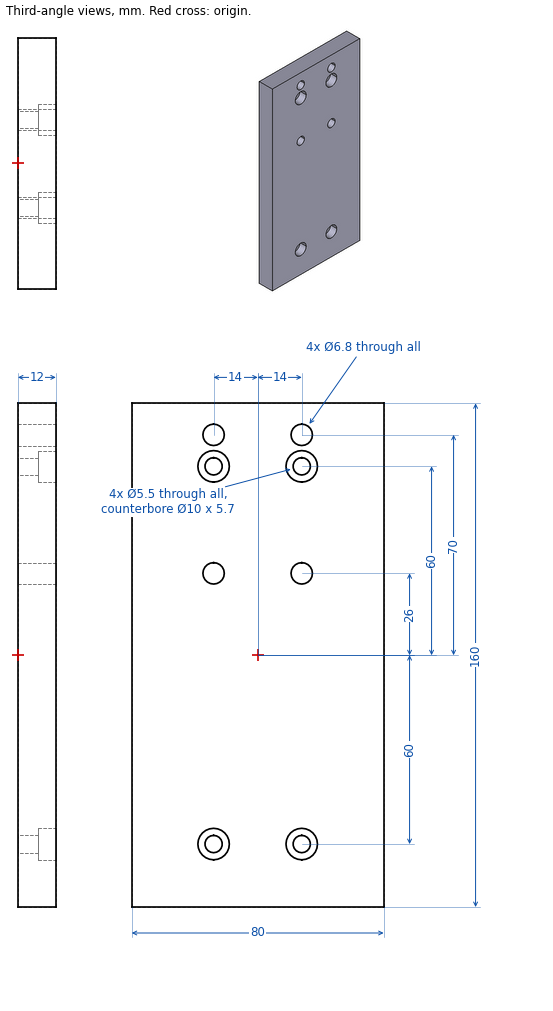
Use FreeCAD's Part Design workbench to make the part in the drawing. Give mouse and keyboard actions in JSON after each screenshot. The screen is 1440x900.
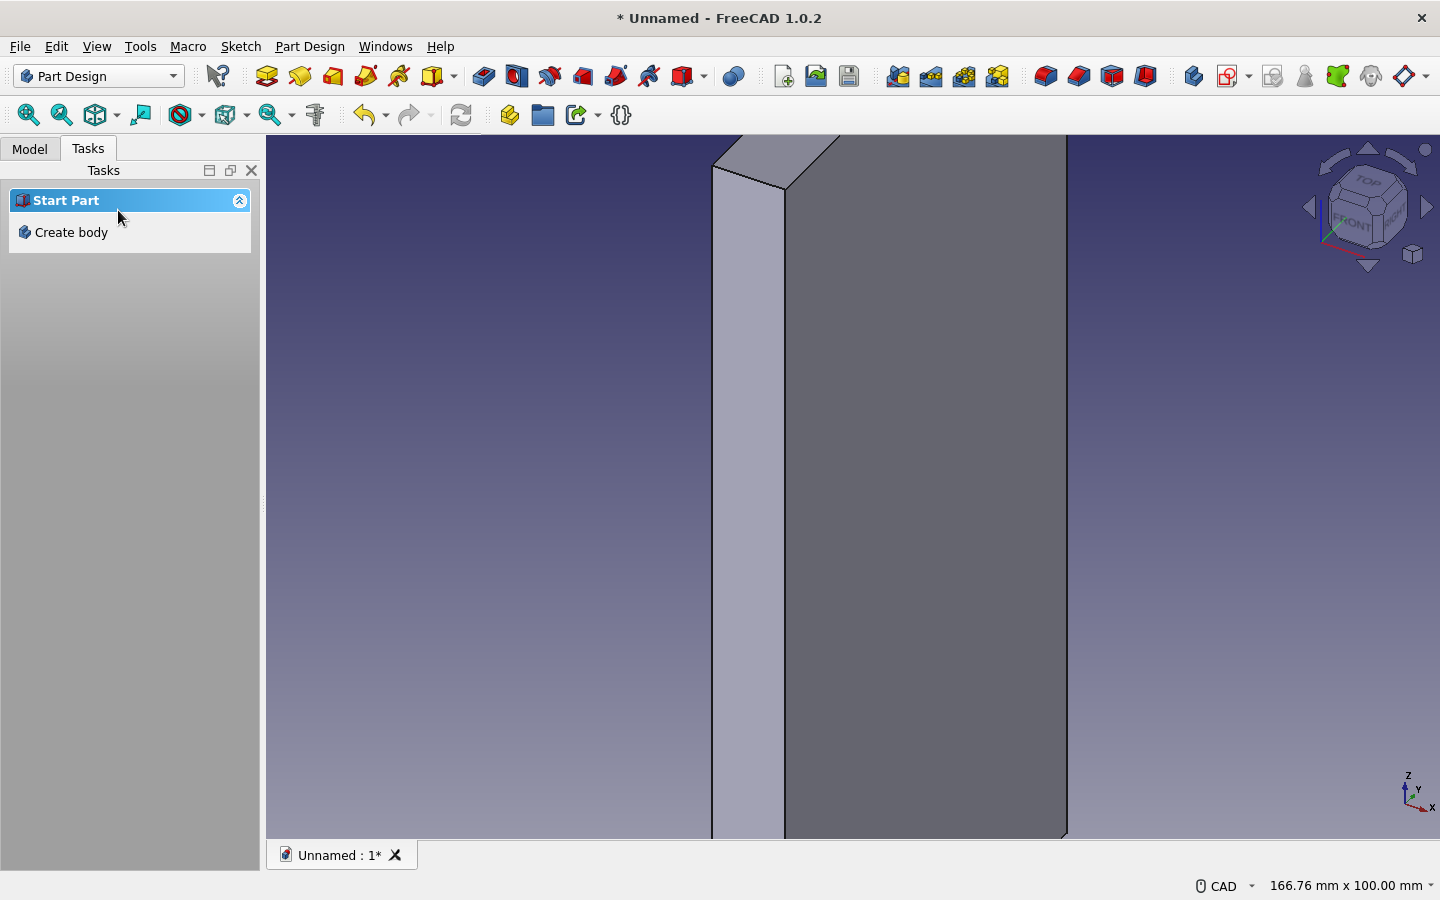
{"action": "left_click", "coordinate": [29, 116]}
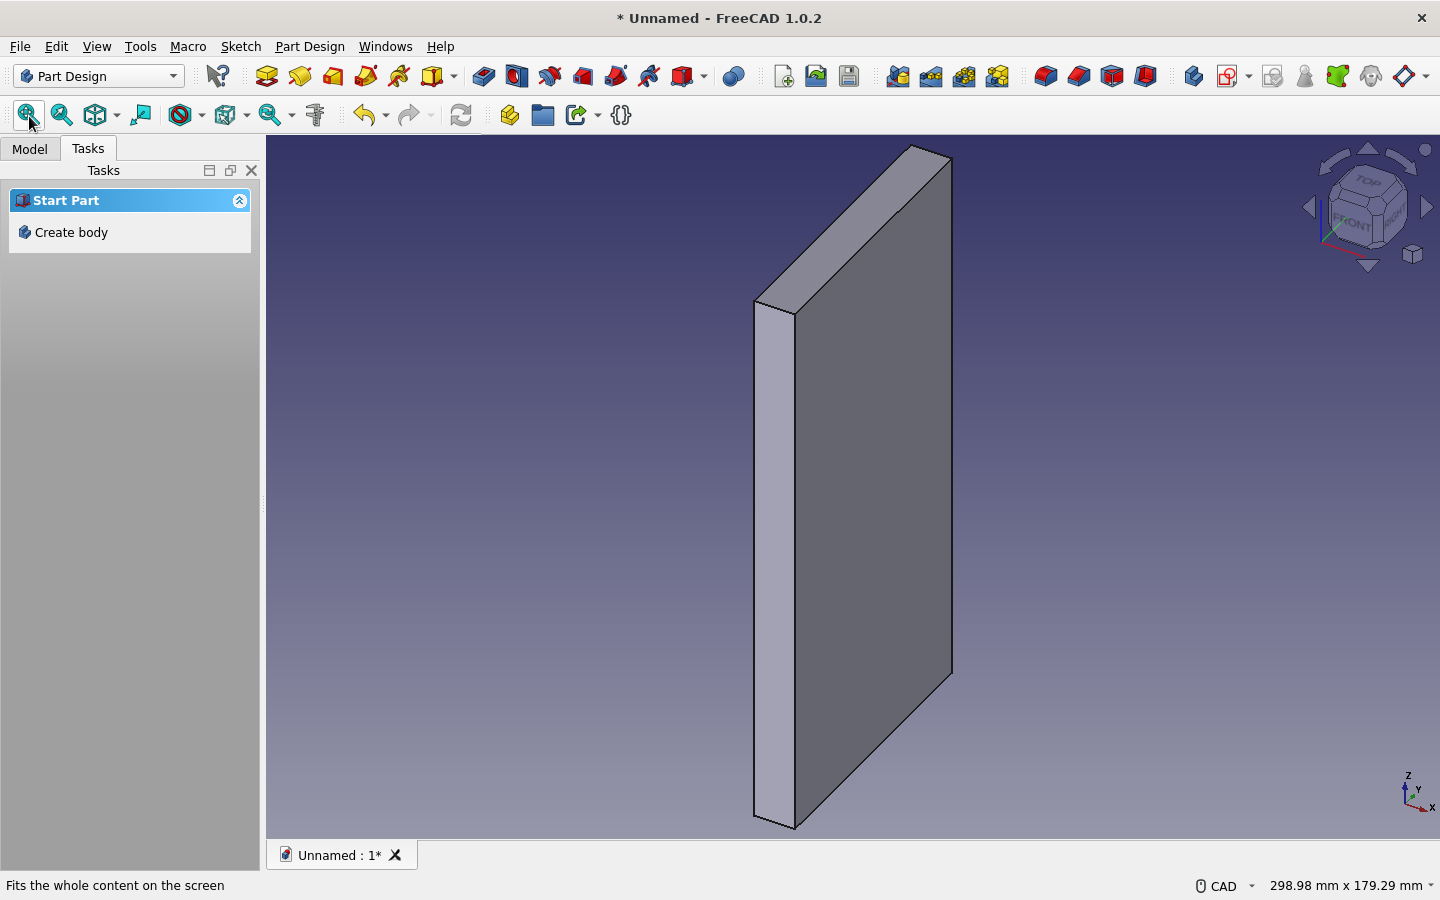
{"action": "left_click", "coordinate": [873, 566]}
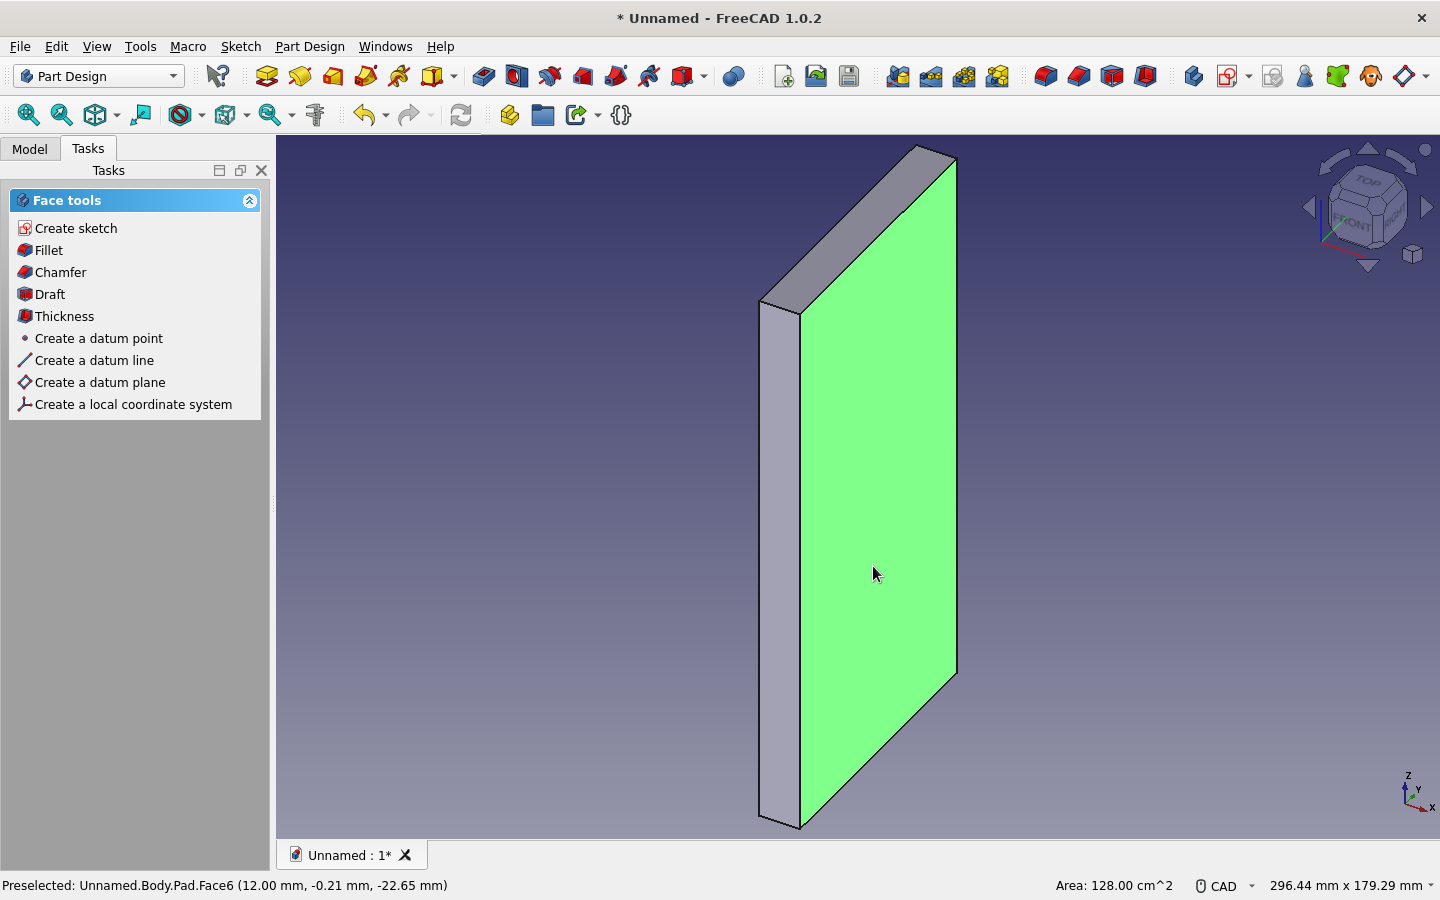
{"action": "left_click", "coordinate": [1226, 76]}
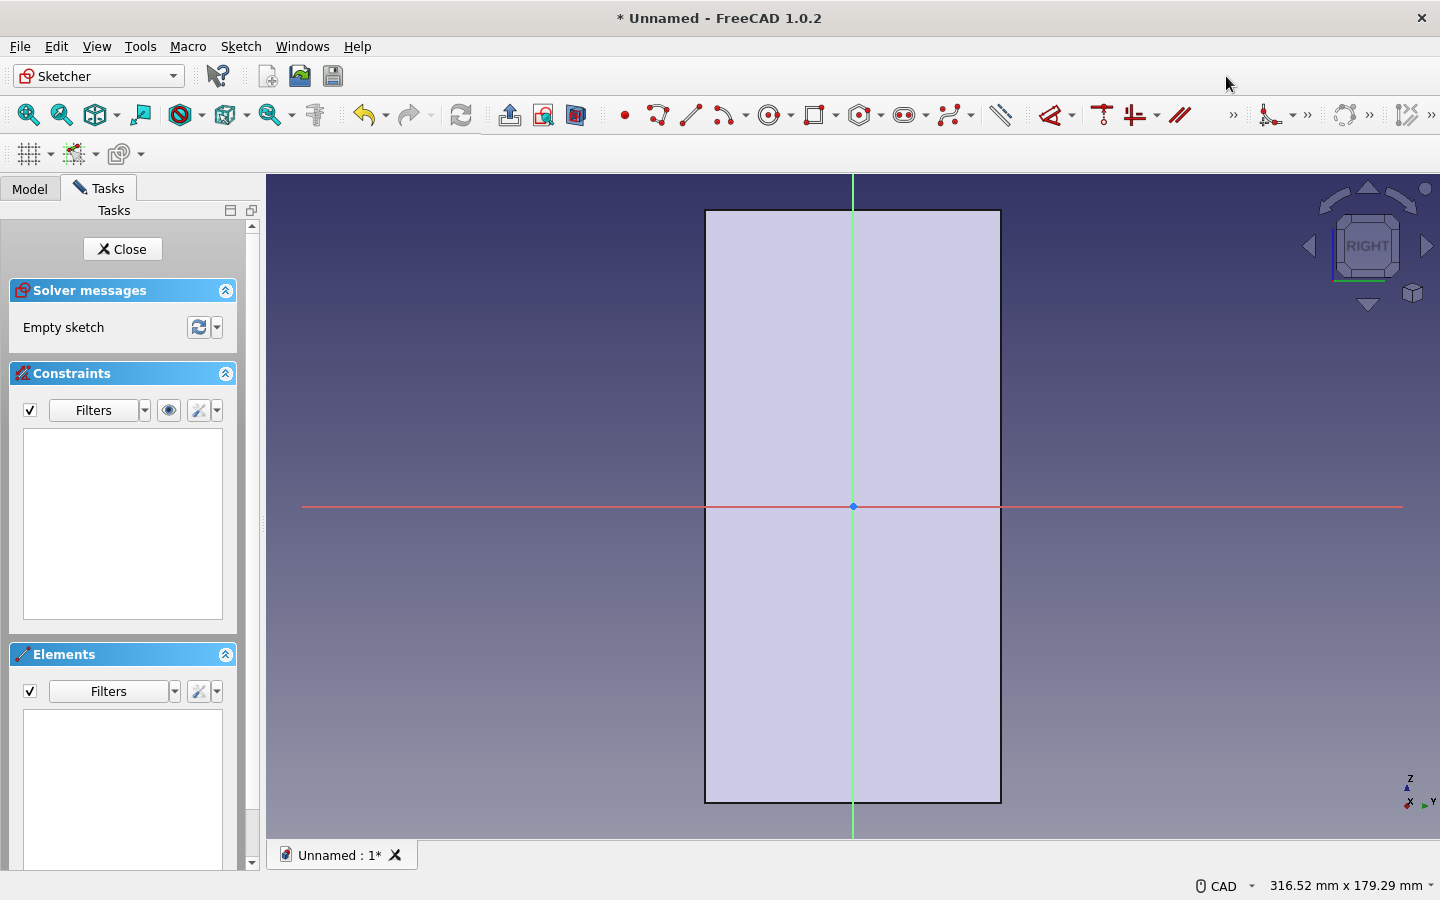
{"action": "scroll", "coordinate": [992, 202], "scroll_direction": "up", "scroll_amount": 2}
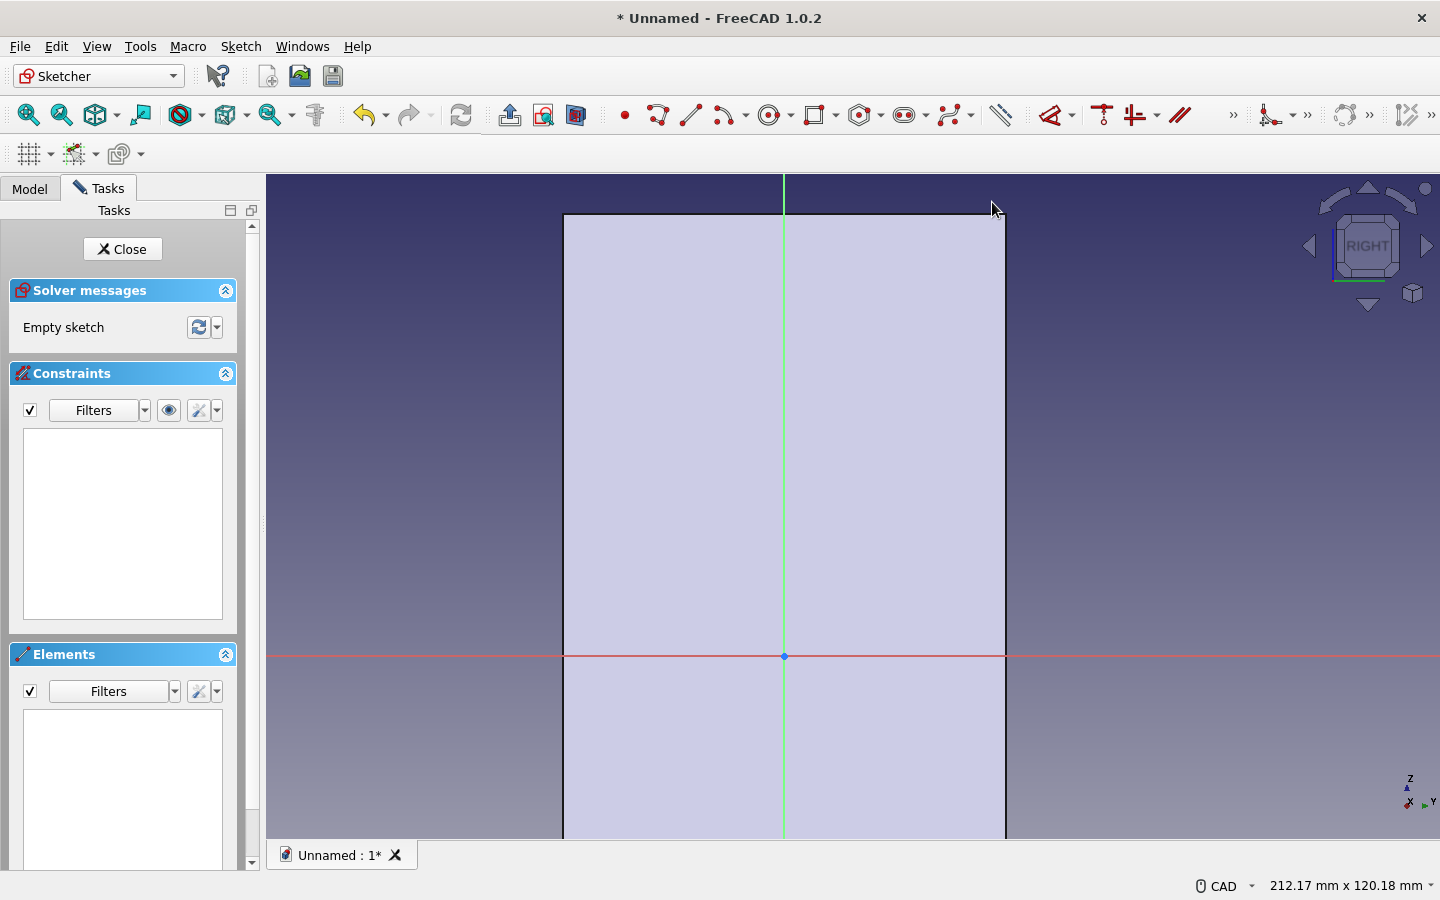
{"action": "left_click", "coordinate": [768, 116]}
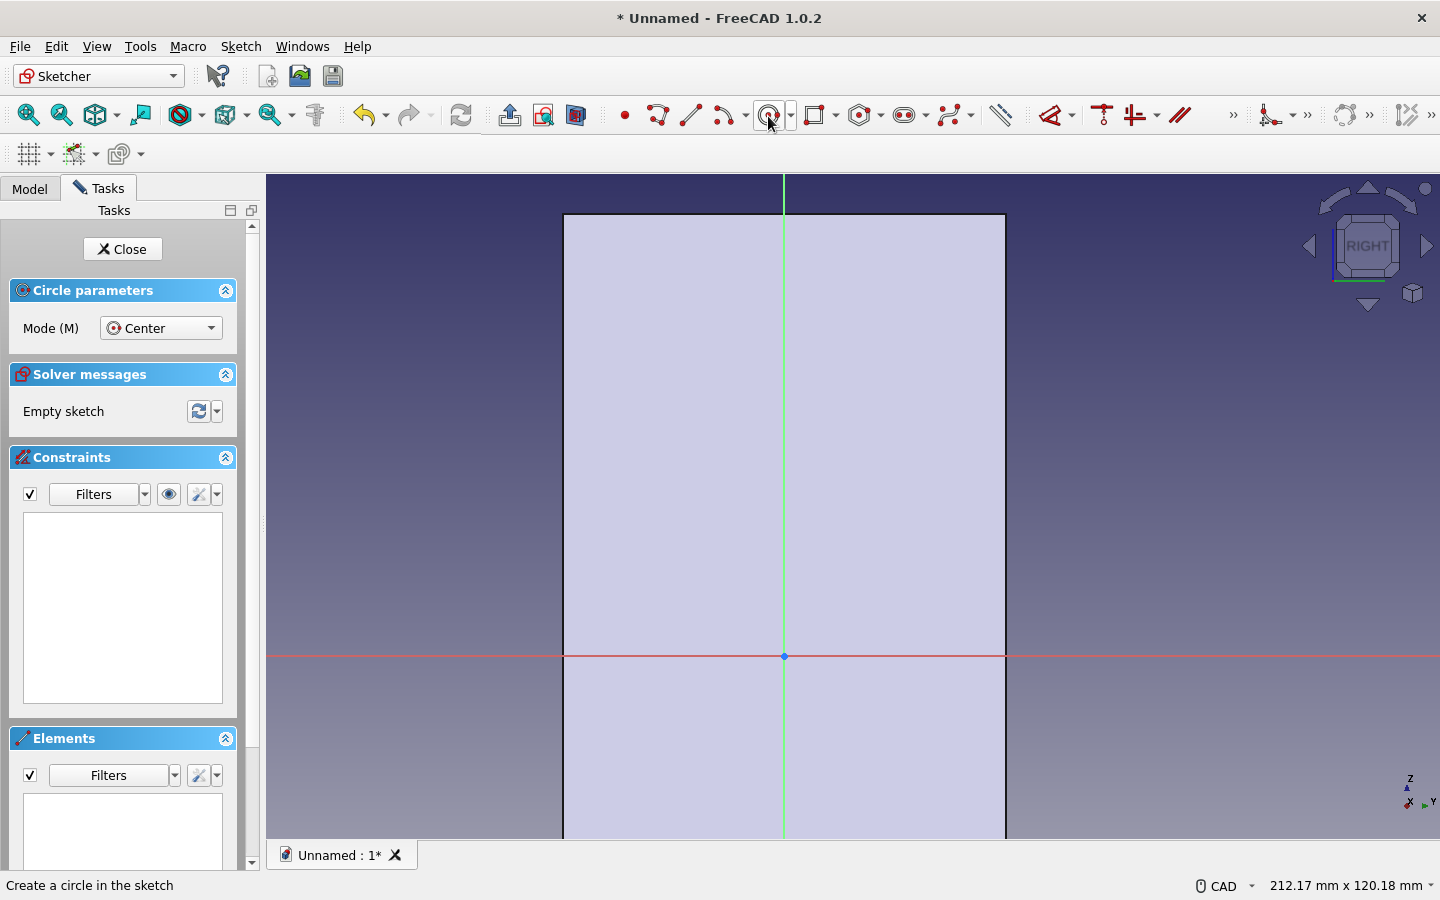
{"action": "left_click", "coordinate": [862, 269]}
{"action": "left_click", "coordinate": [875, 256]}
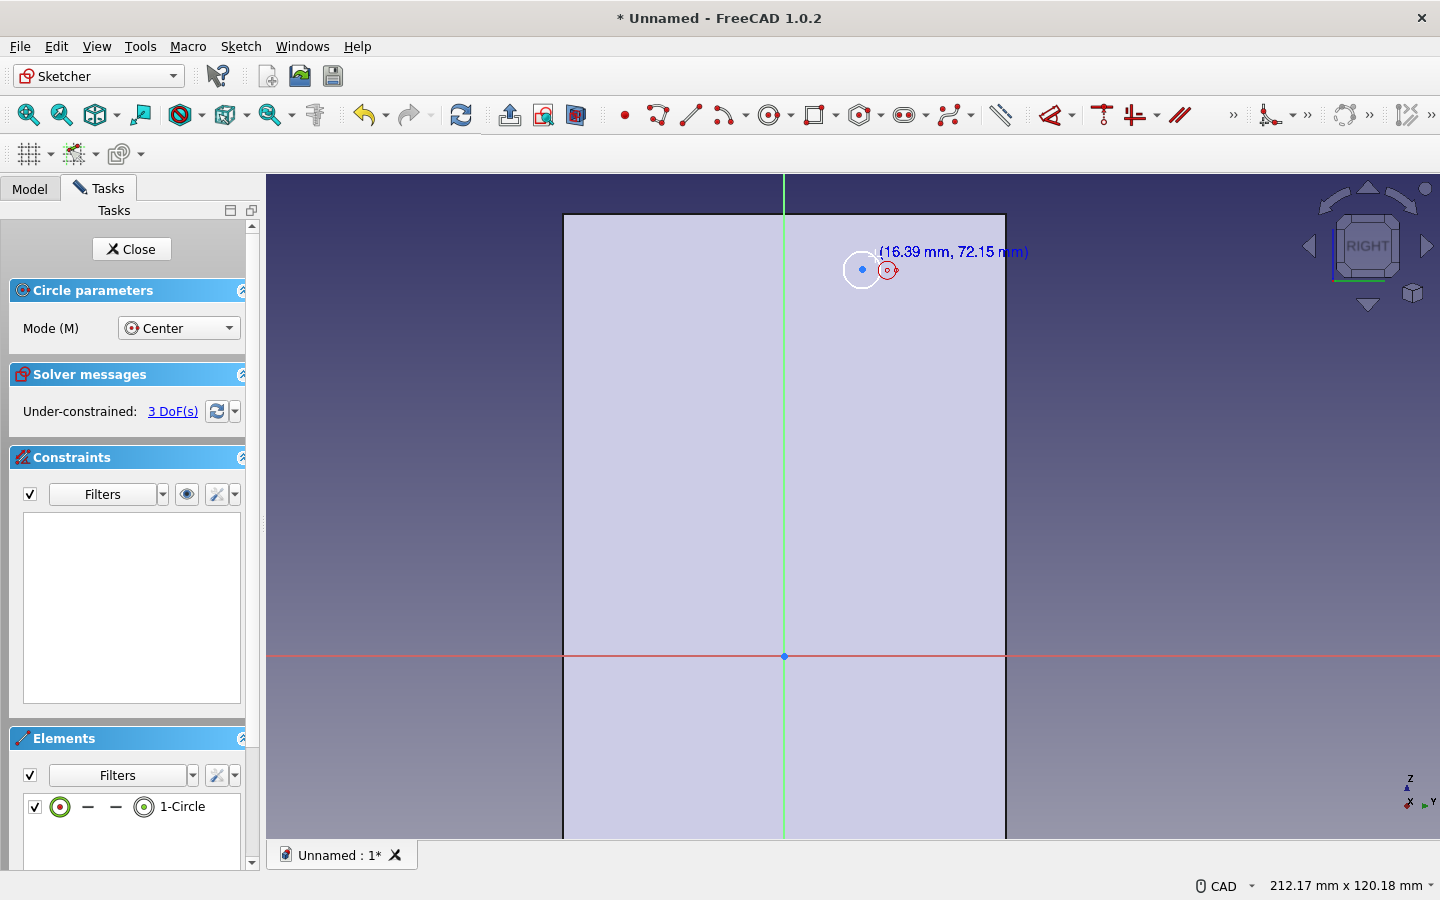
{"action": "left_click", "coordinate": [707, 269]}
{"action": "left_click", "coordinate": [720, 256]}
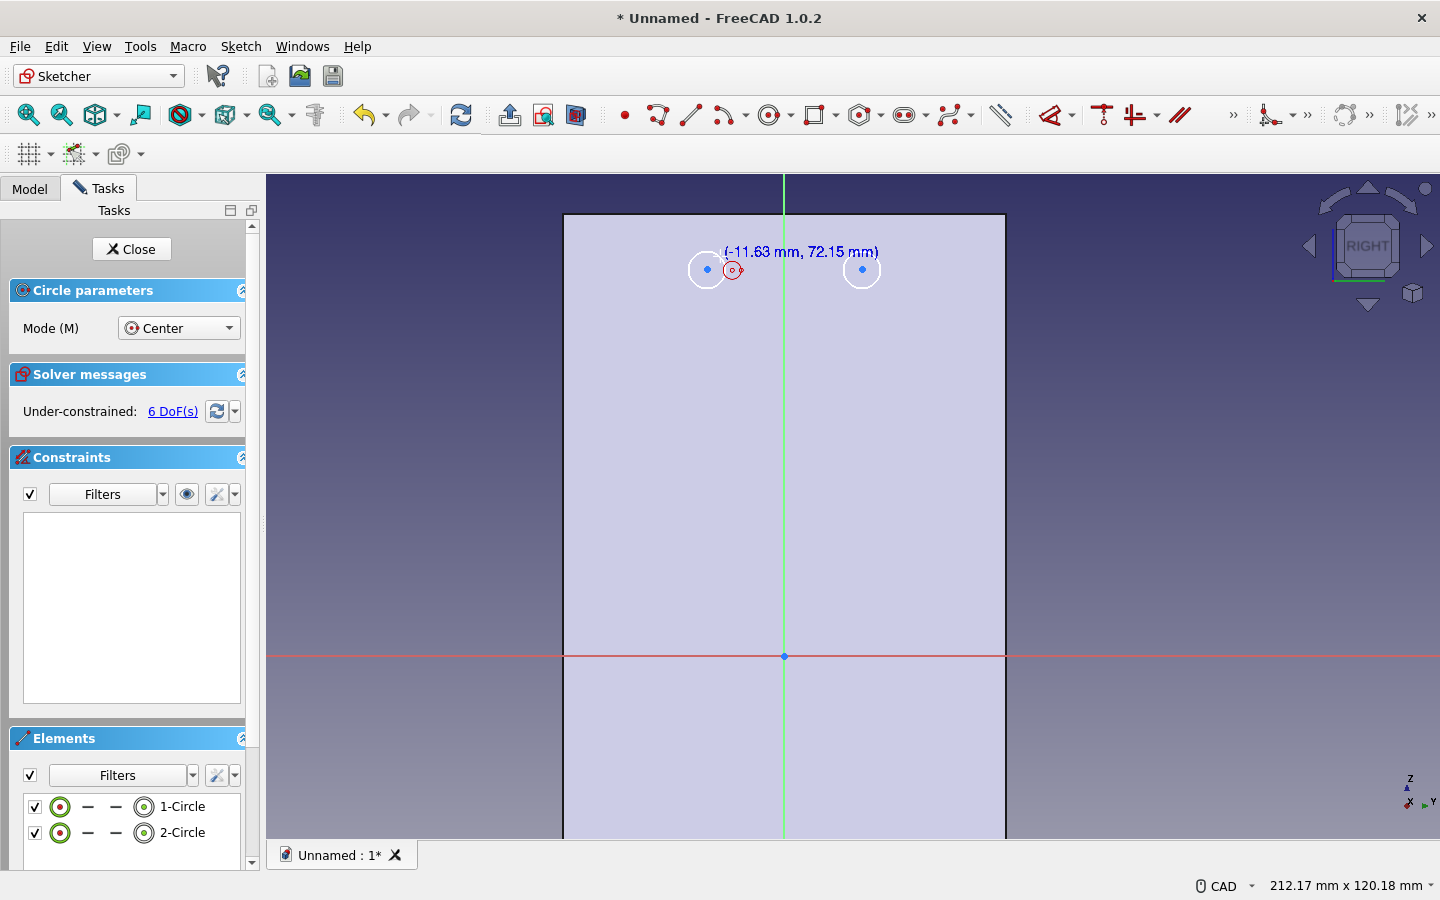
{"action": "left_click", "coordinate": [862, 512]}
{"action": "left_click", "coordinate": [875, 499]}